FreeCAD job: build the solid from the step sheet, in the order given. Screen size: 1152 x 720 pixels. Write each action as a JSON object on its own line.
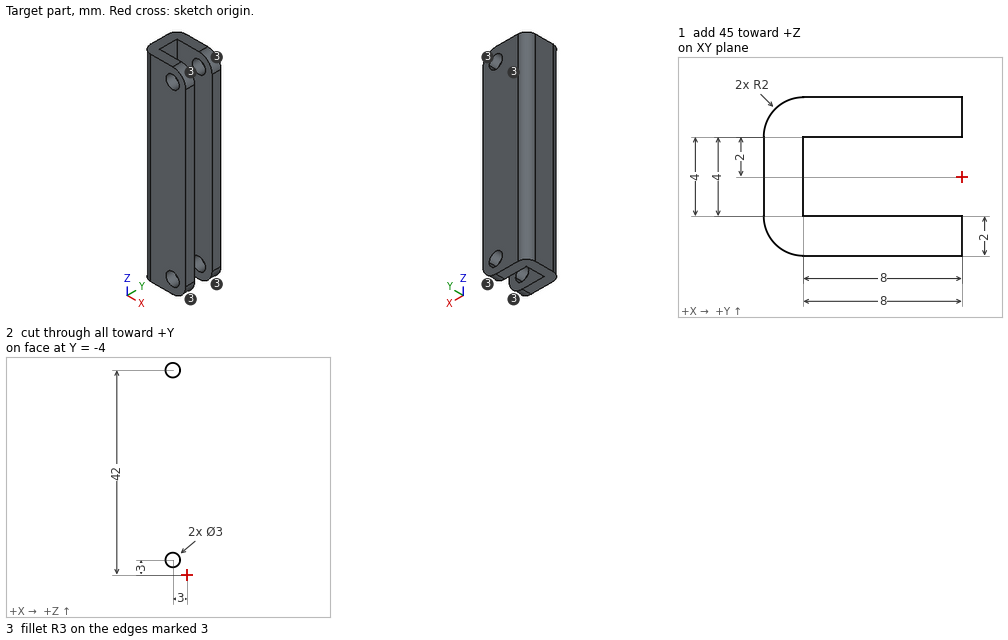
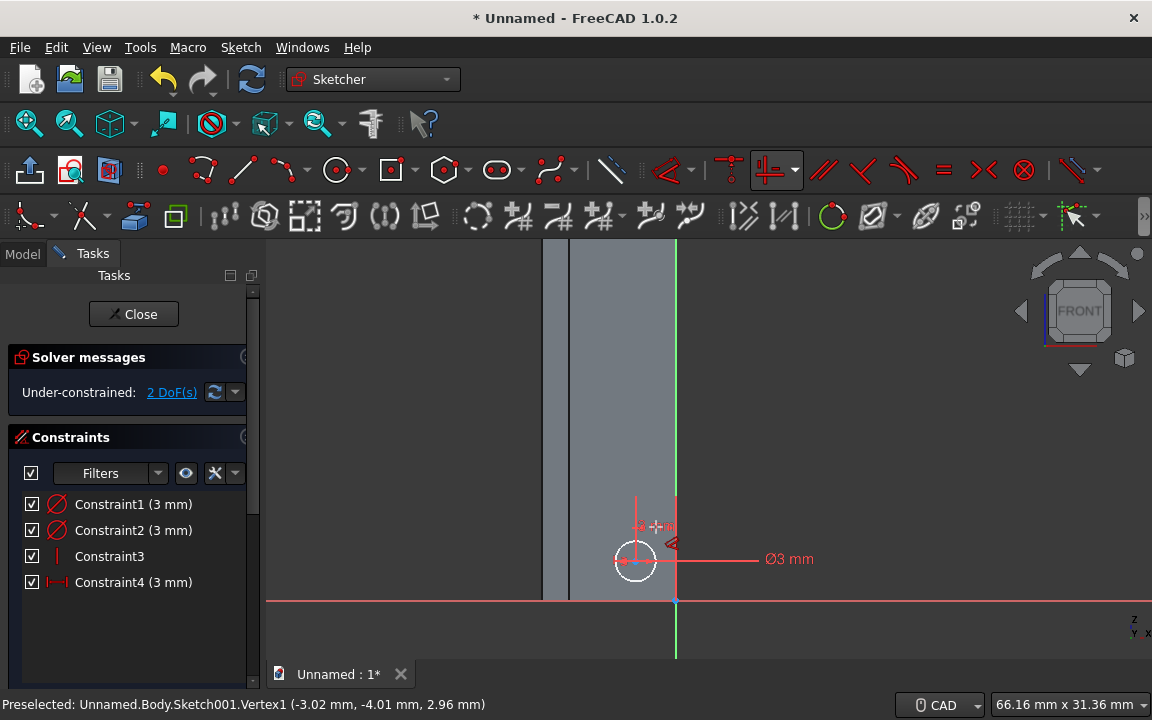
{"action": "left_click", "coordinate": [636, 561]}
{"action": "left_click", "coordinate": [710, 581]}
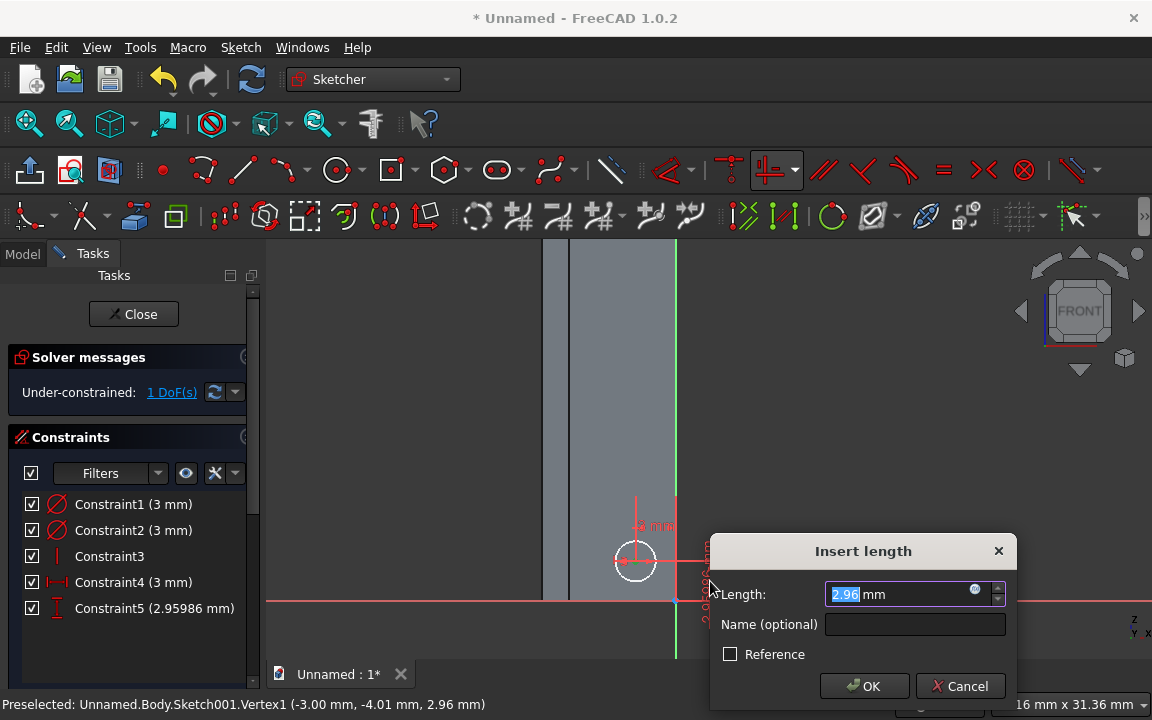
{"action": "type", "text": "3"}
{"action": "key", "text": "Return"}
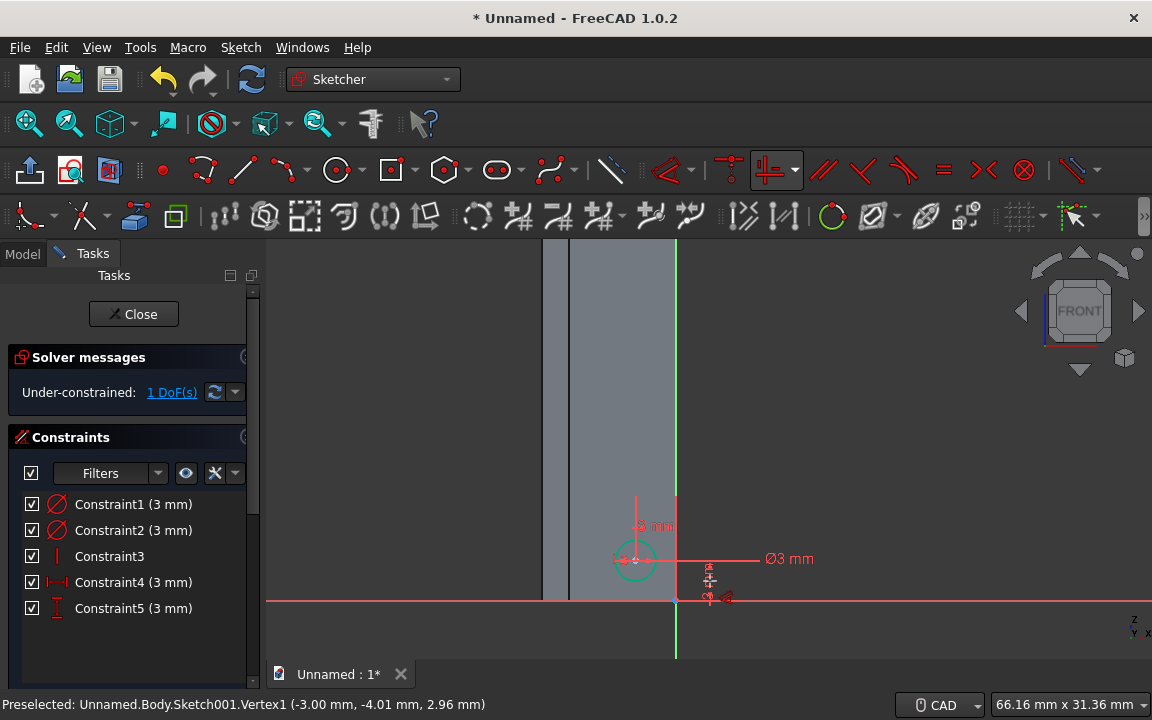
{"action": "scroll", "coordinate": [636, 563], "scroll_direction": "down", "scroll_amount": 4}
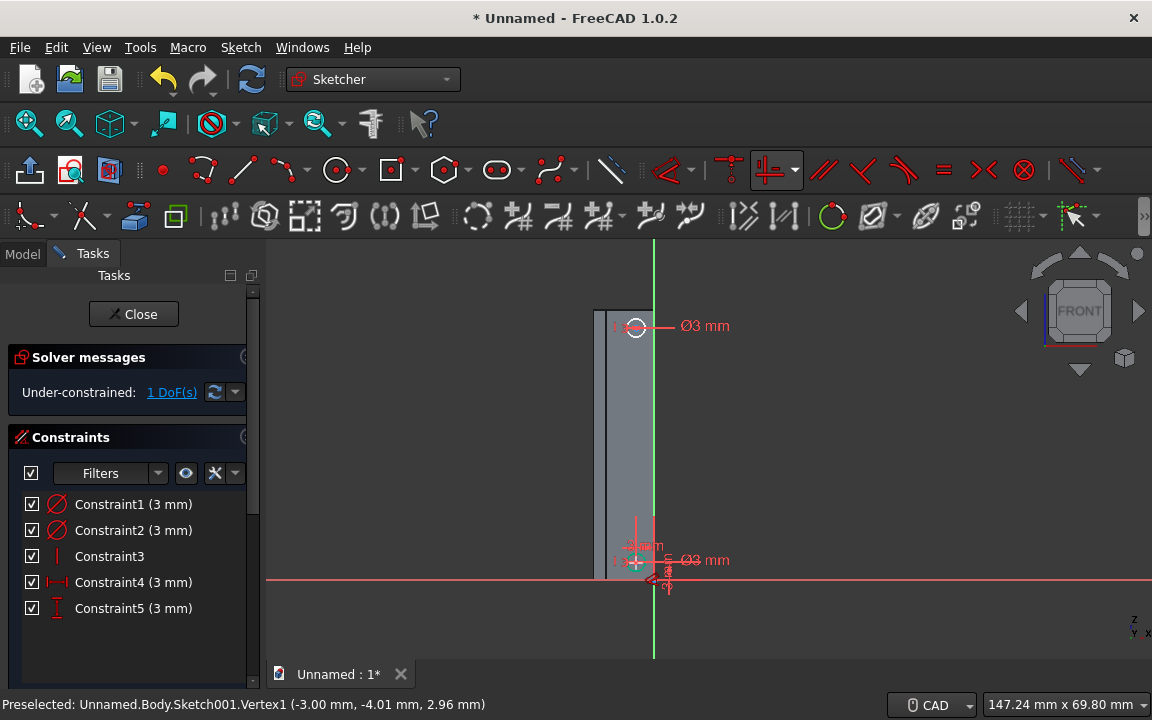
{"action": "left_click", "coordinate": [636, 328]}
{"action": "left_click", "coordinate": [688, 454]}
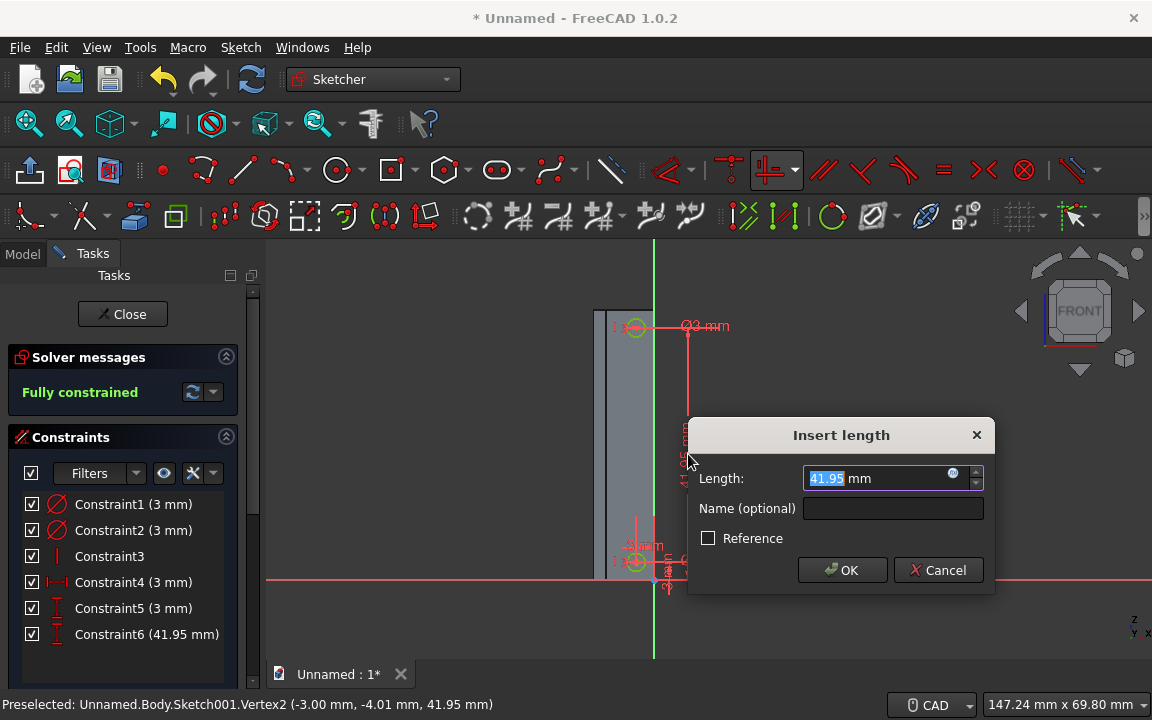
{"action": "type", "text": "42"}
{"action": "key", "text": "Return"}
{"action": "key", "text": "Escape"}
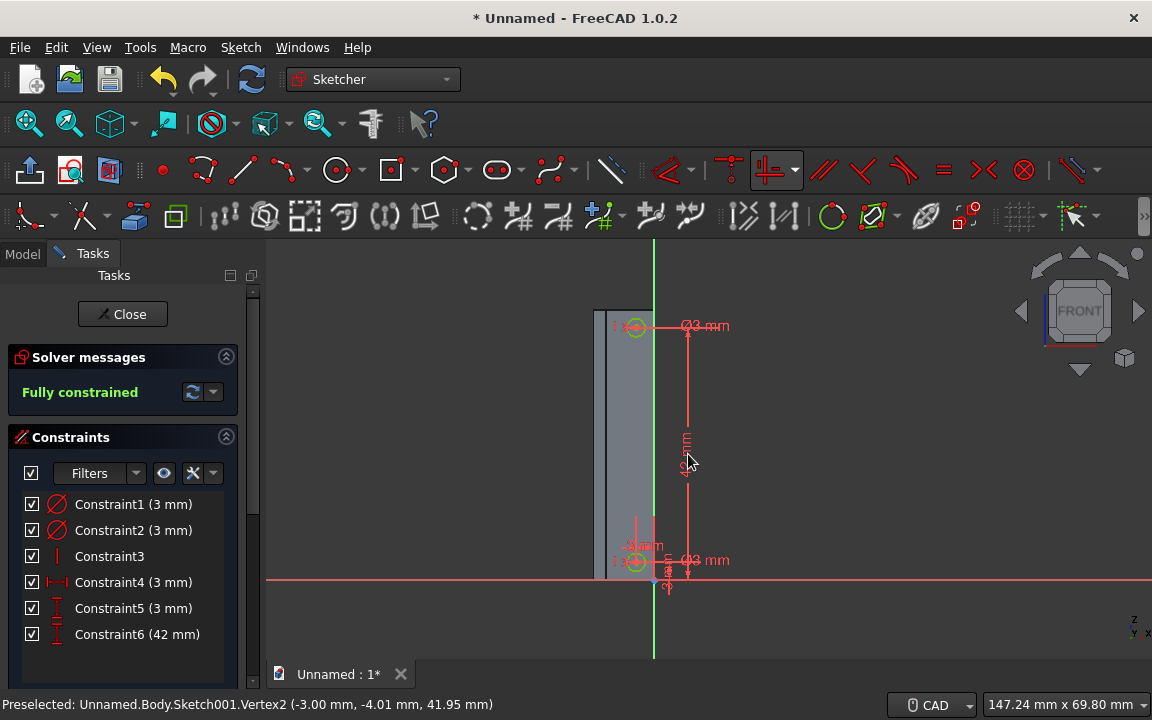
{"action": "left_click", "coordinate": [123, 314]}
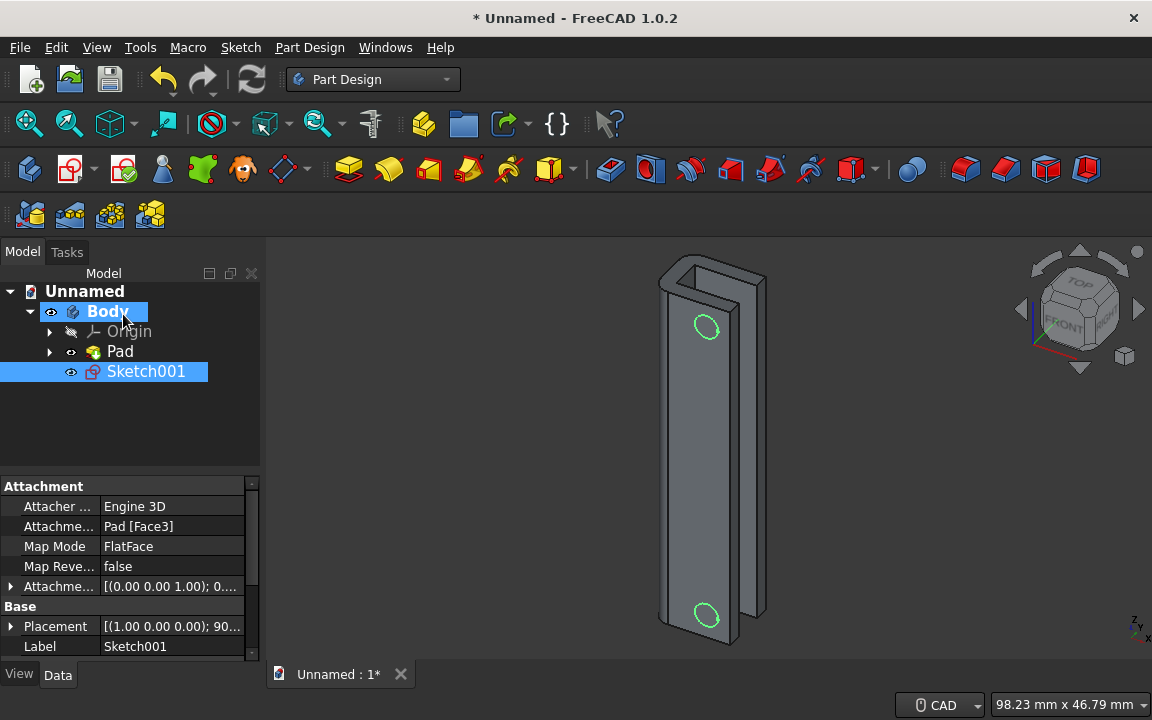
{"action": "left_click", "coordinate": [612, 170]}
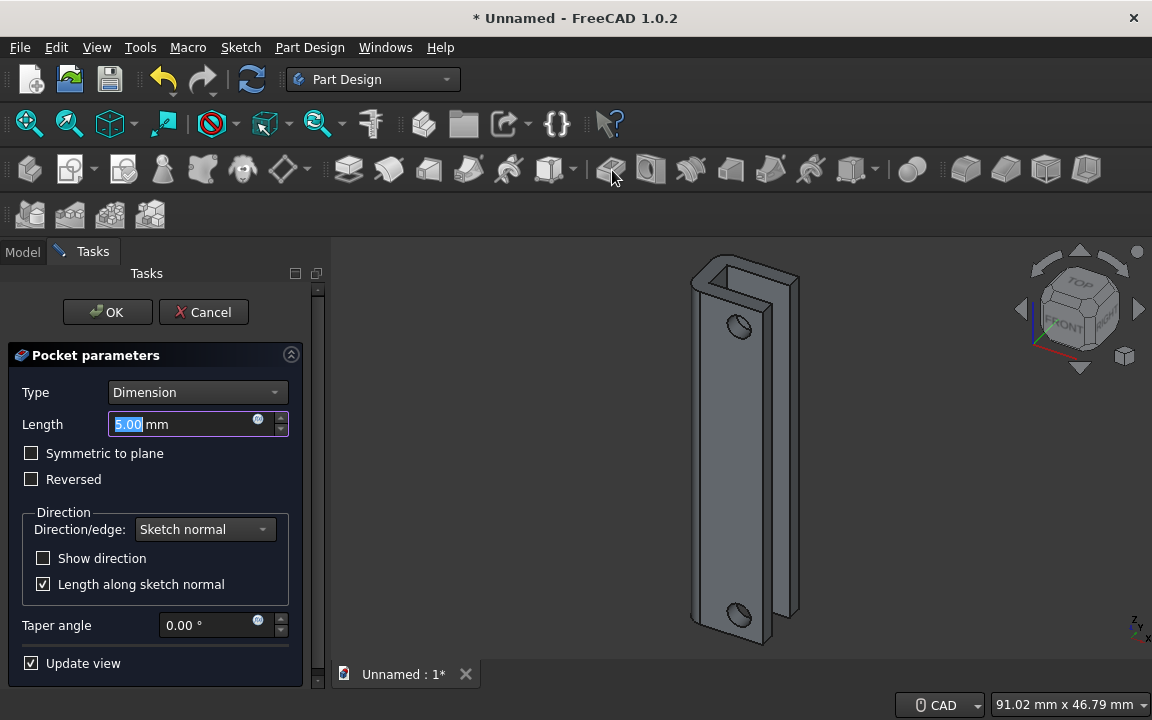
{"action": "left_click", "coordinate": [198, 392]}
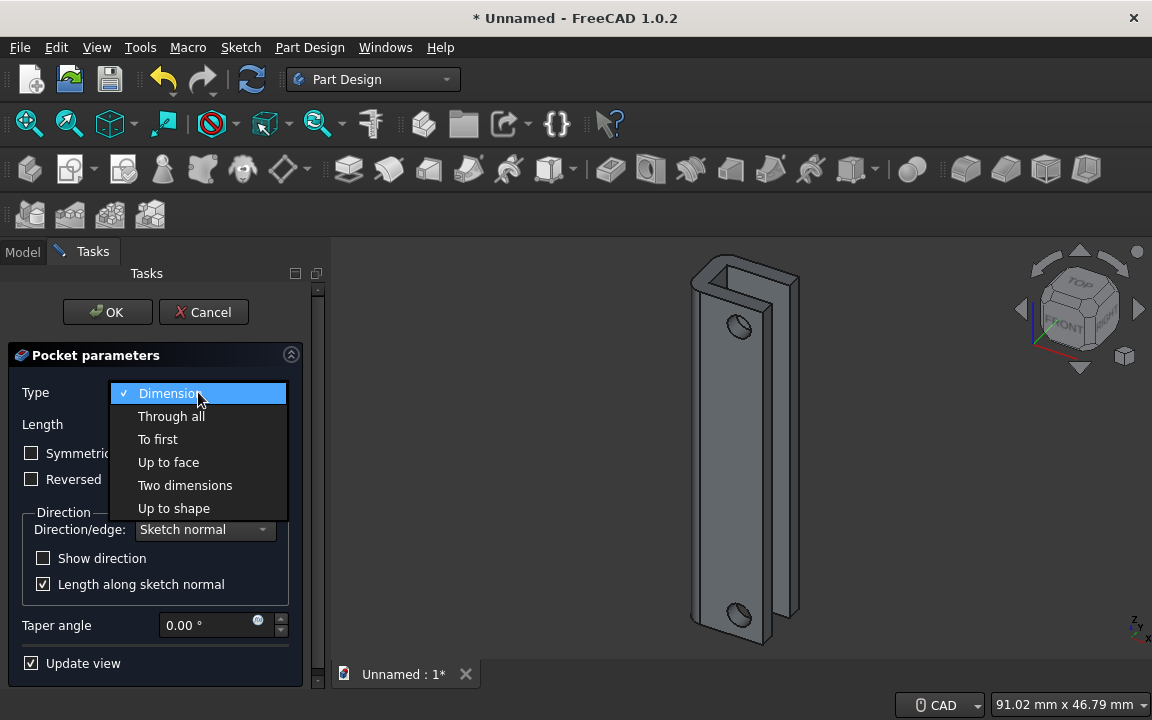
{"action": "left_click", "coordinate": [198, 416]}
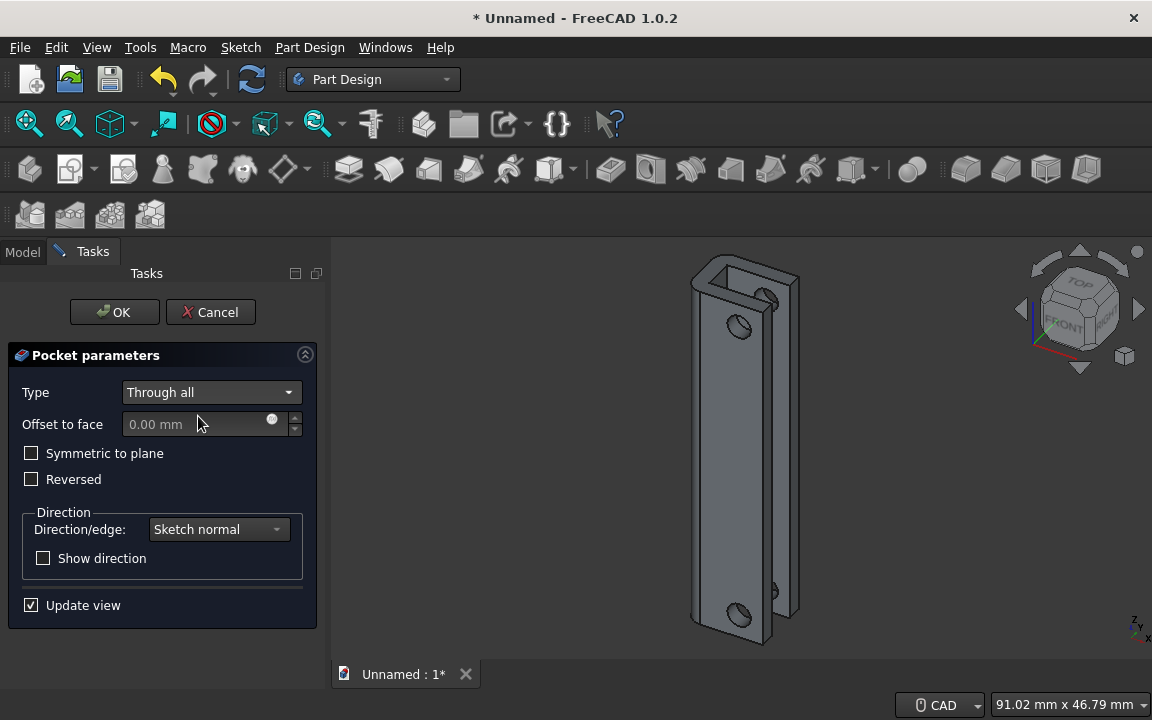
{"action": "left_click", "coordinate": [115, 312]}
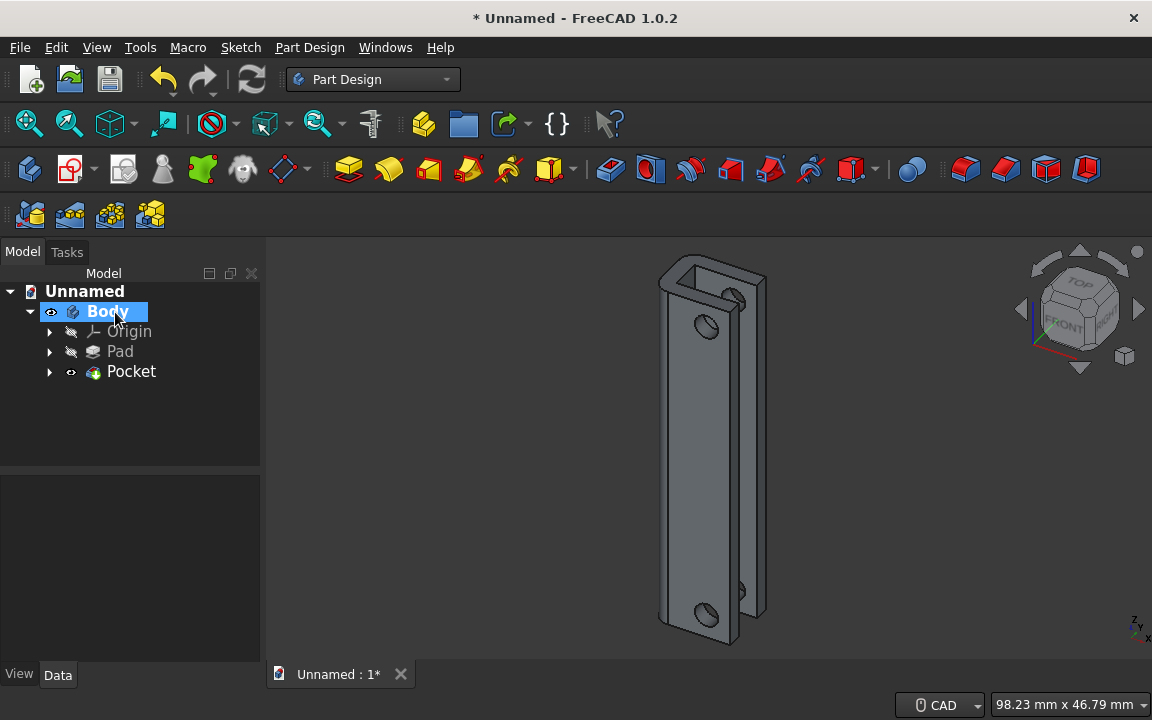
{"action": "left_click", "coordinate": [762, 280]}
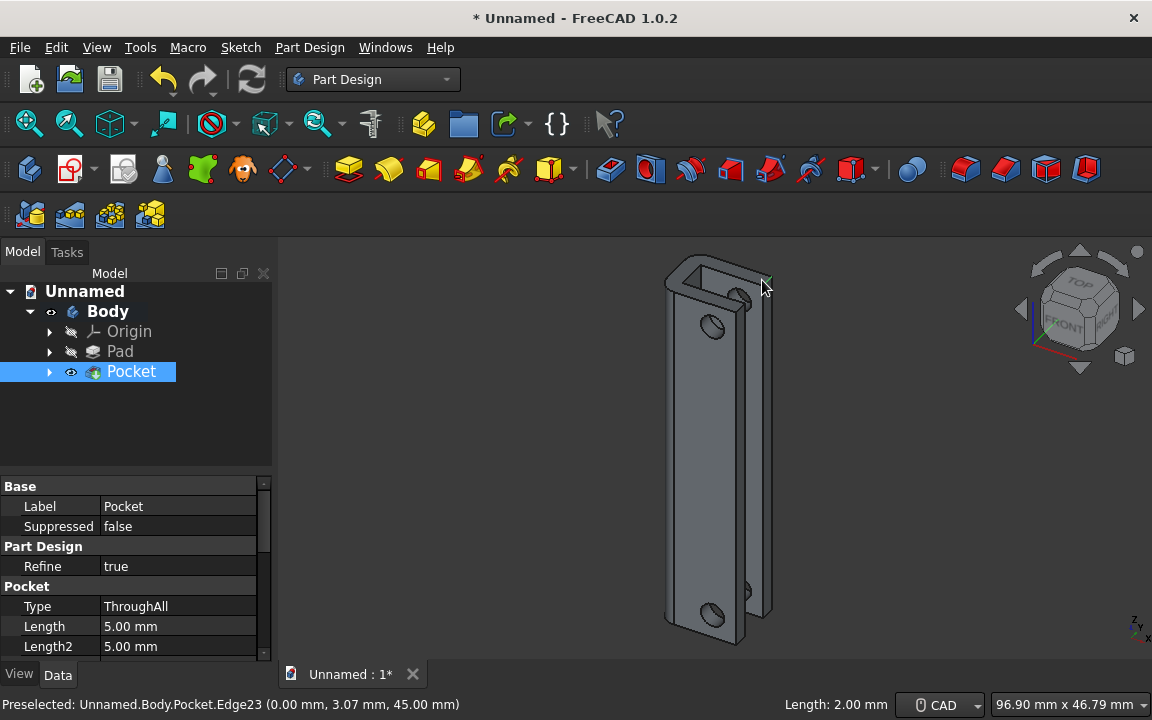
{"action": "left_click", "coordinate": [741, 307], "text": "ctrl"}